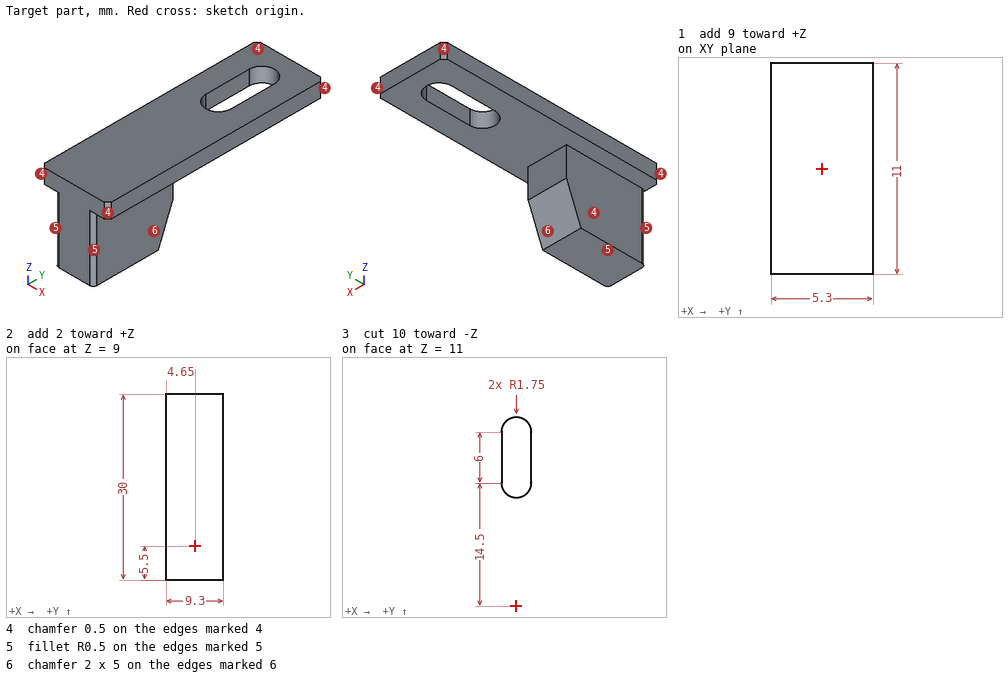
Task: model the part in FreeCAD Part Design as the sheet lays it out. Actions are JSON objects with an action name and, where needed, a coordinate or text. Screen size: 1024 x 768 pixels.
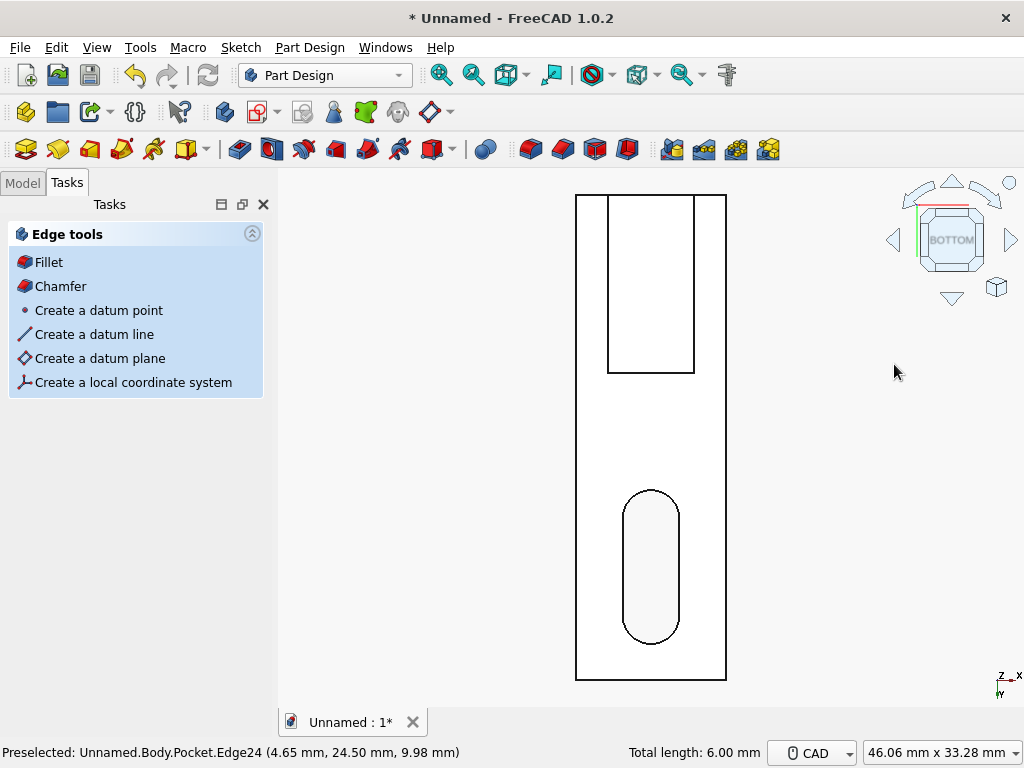
{"action": "key", "text": "4"}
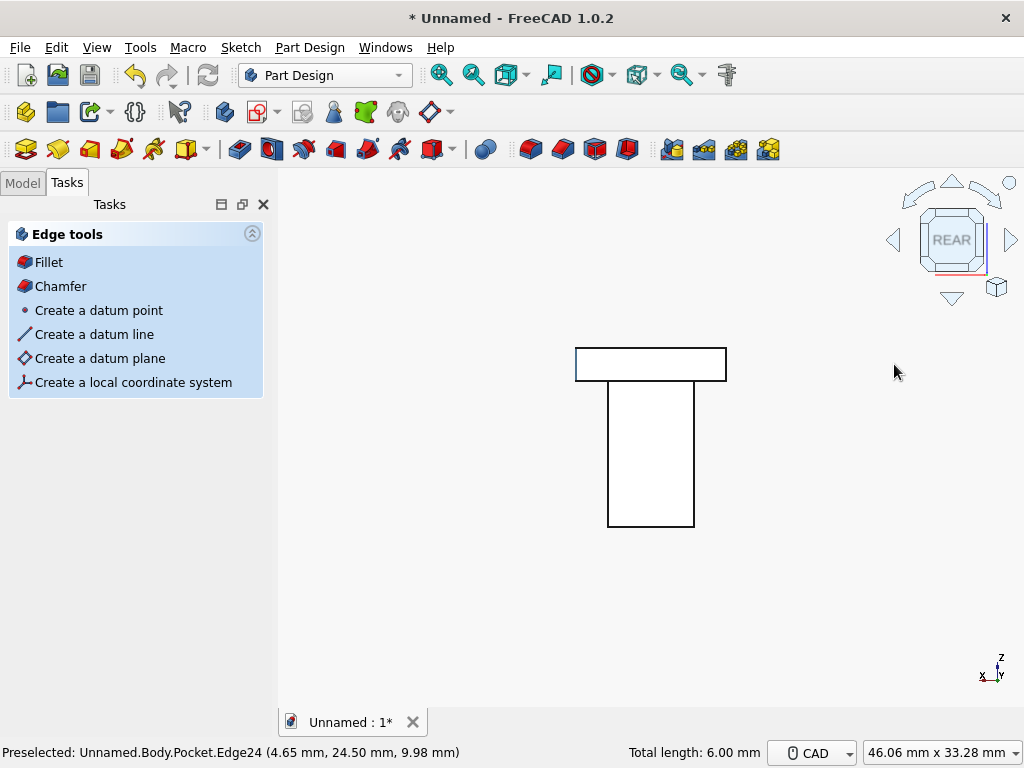
{"action": "left_click", "coordinate": [442, 76]}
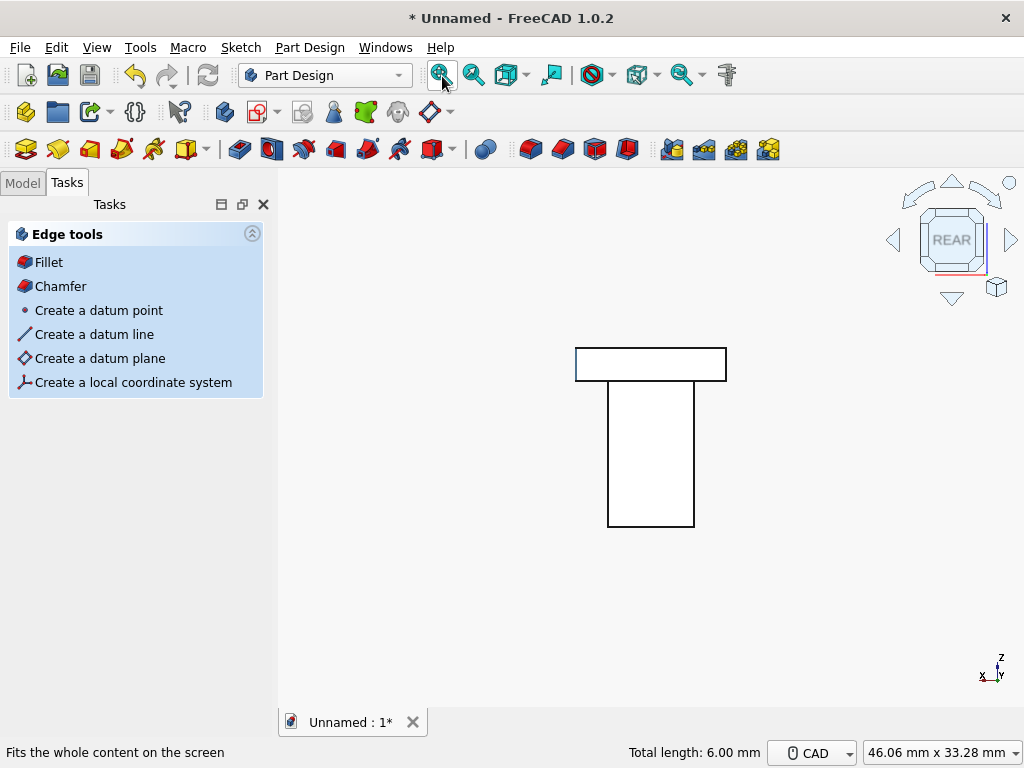
{"action": "left_click", "coordinate": [726, 364], "text": "ctrl"}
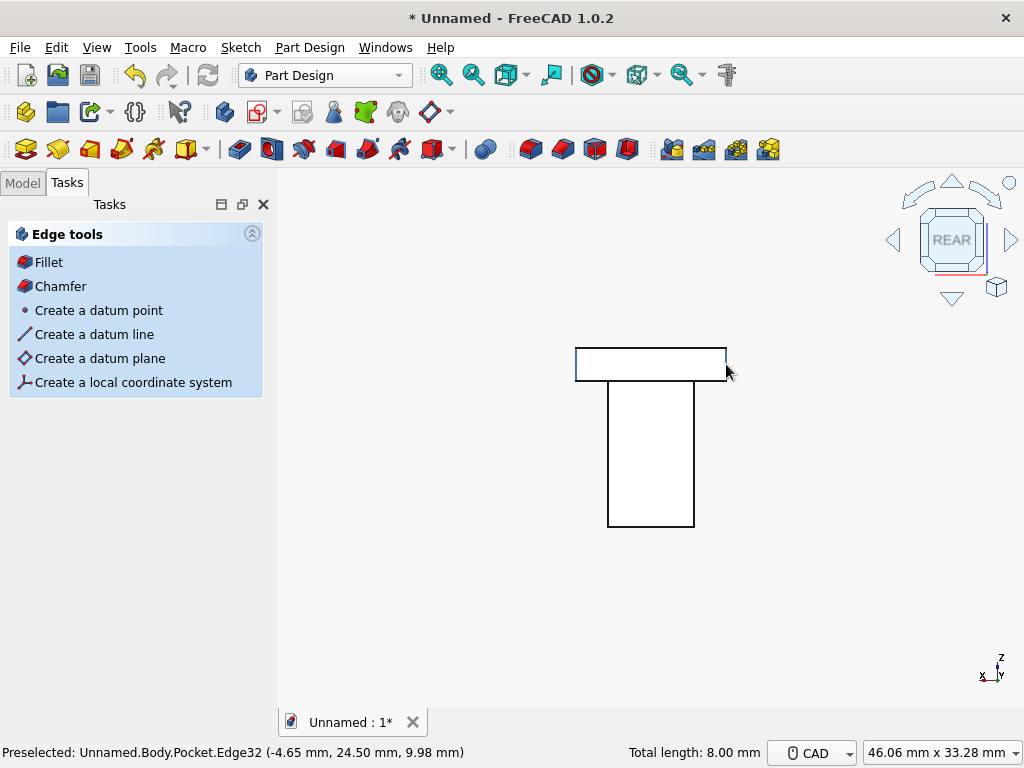
{"action": "left_click", "coordinate": [564, 150]}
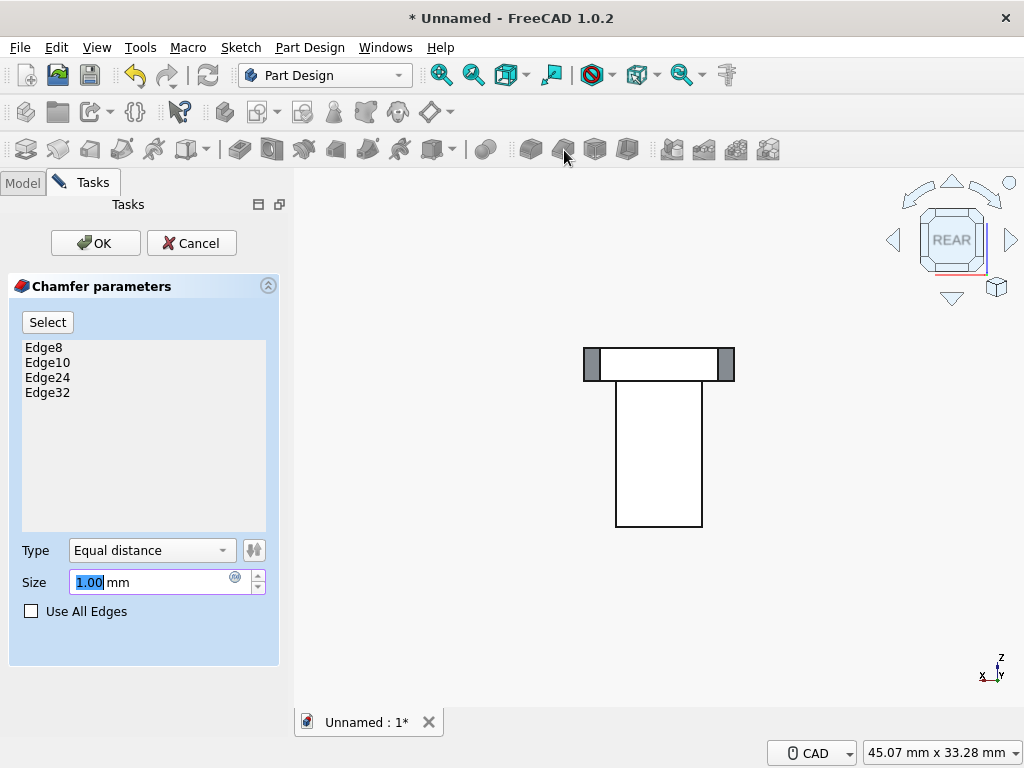
{"action": "type", "text": "0.5"}
{"action": "key", "text": "Tab"}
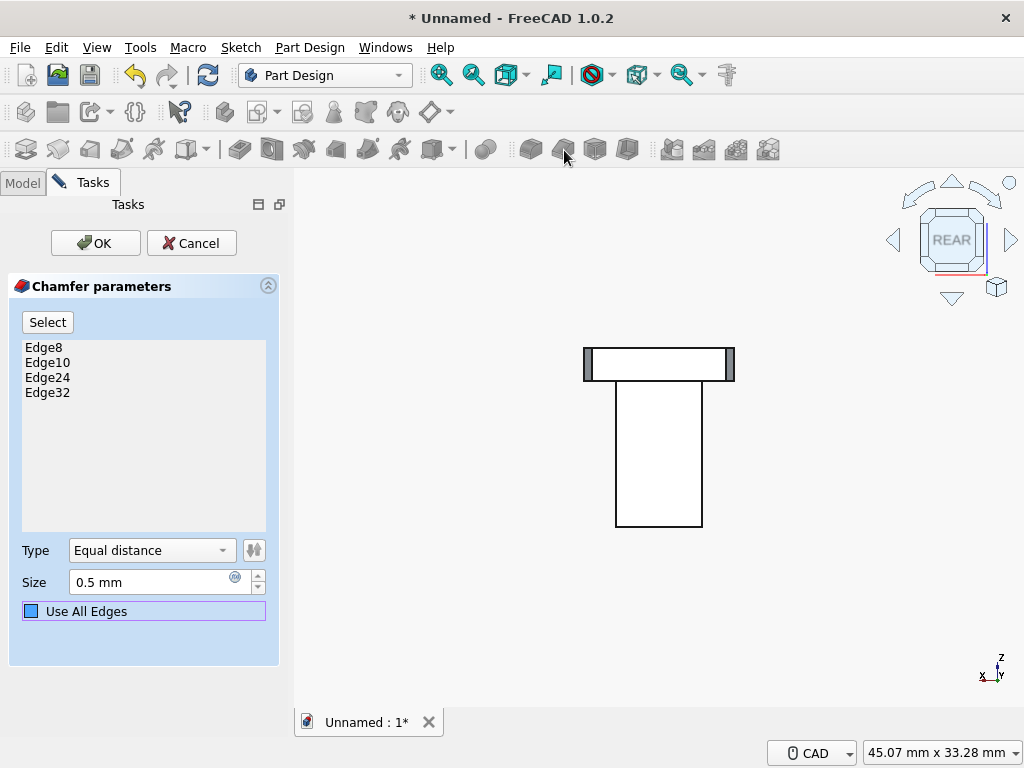
{"action": "left_click", "coordinate": [96, 243]}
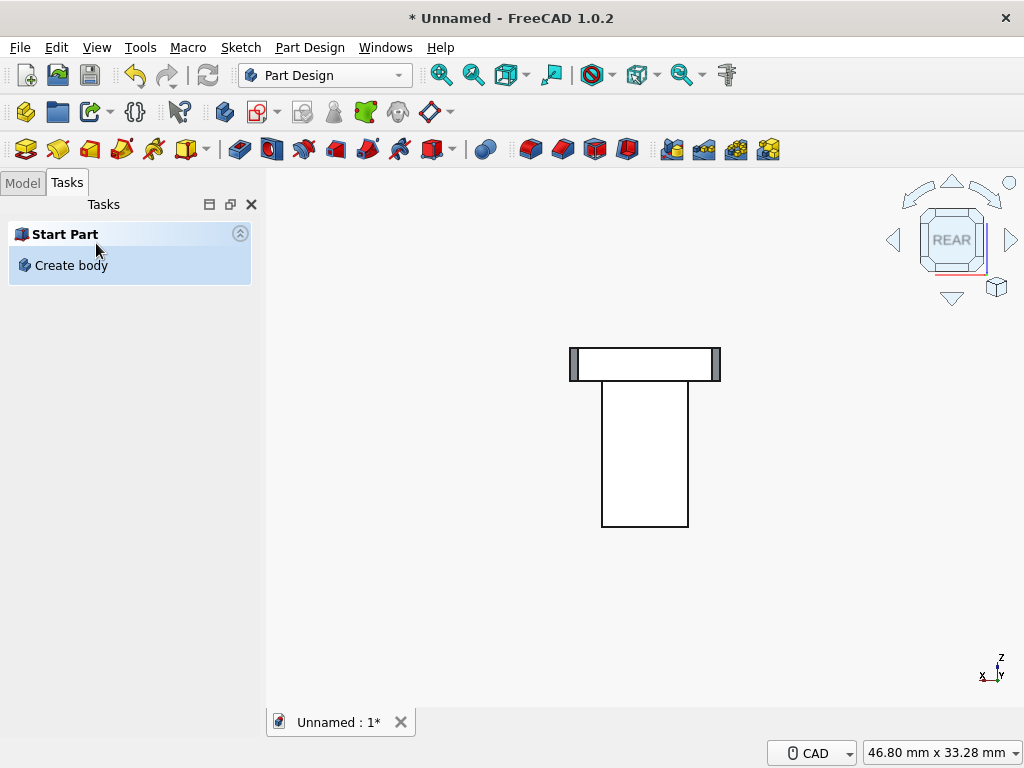
{"action": "left_click", "coordinate": [442, 76]}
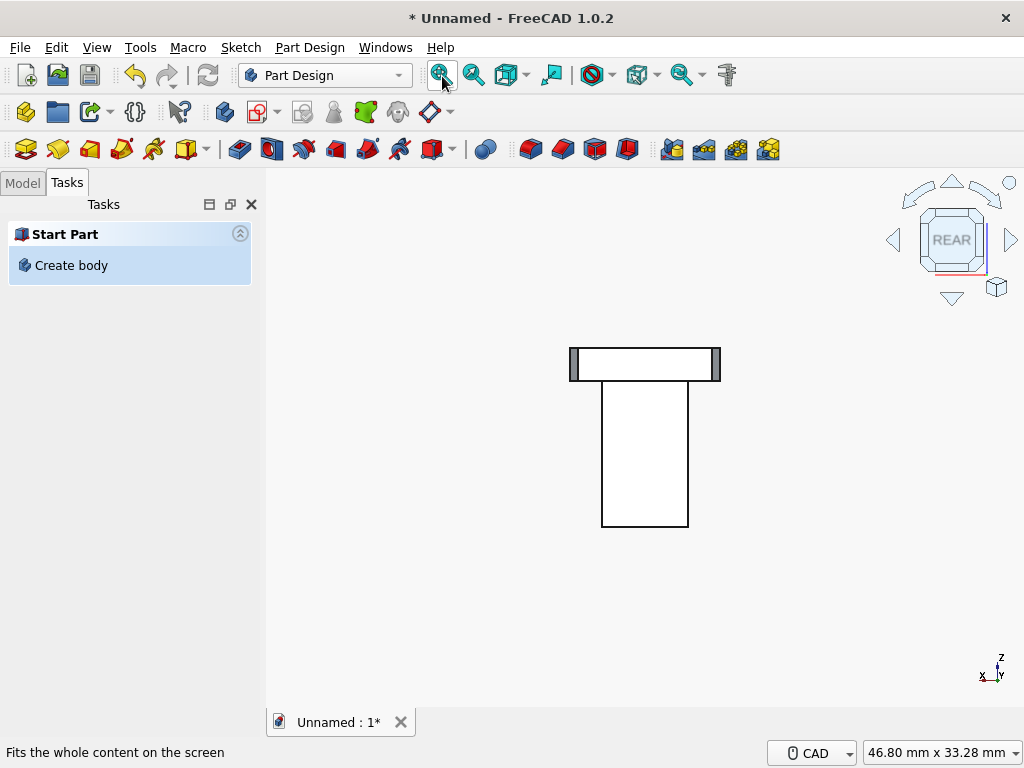
{"action": "key", "text": "0"}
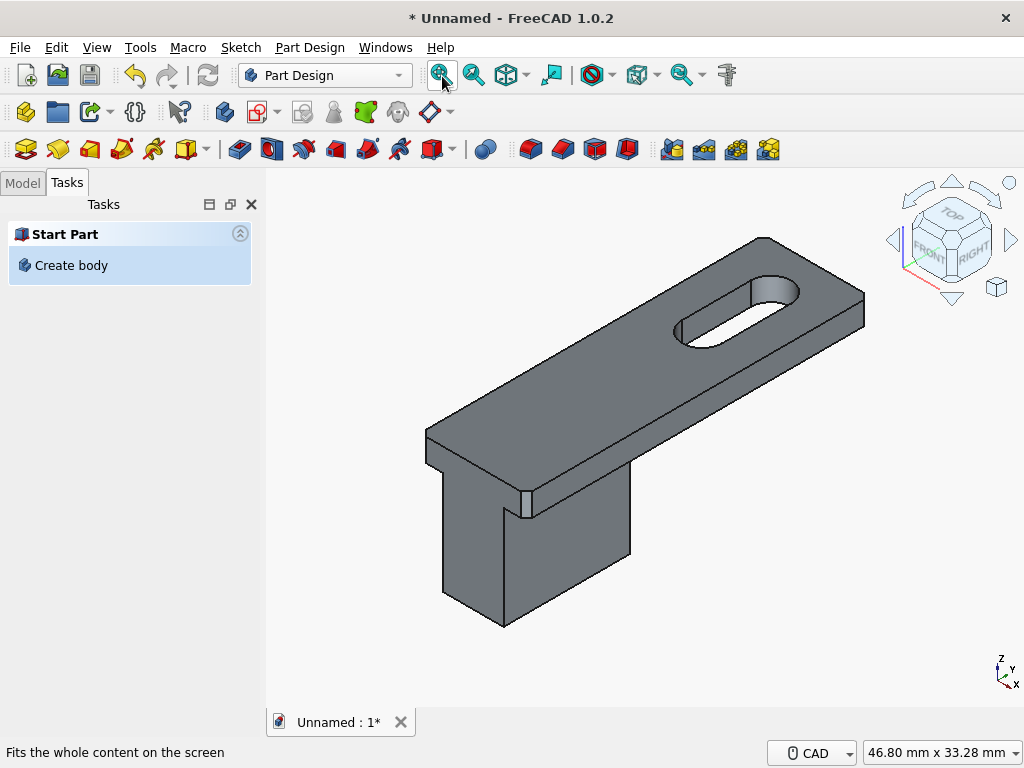
{"action": "left_click", "coordinate": [504, 566]}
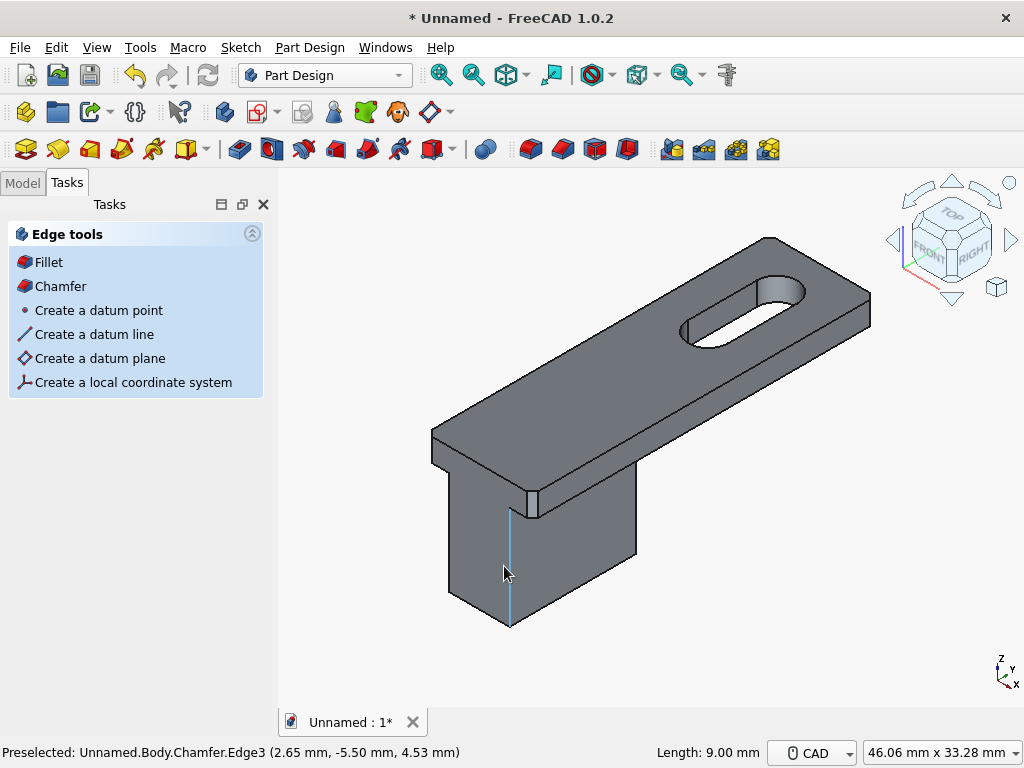
{"action": "key", "text": "2"}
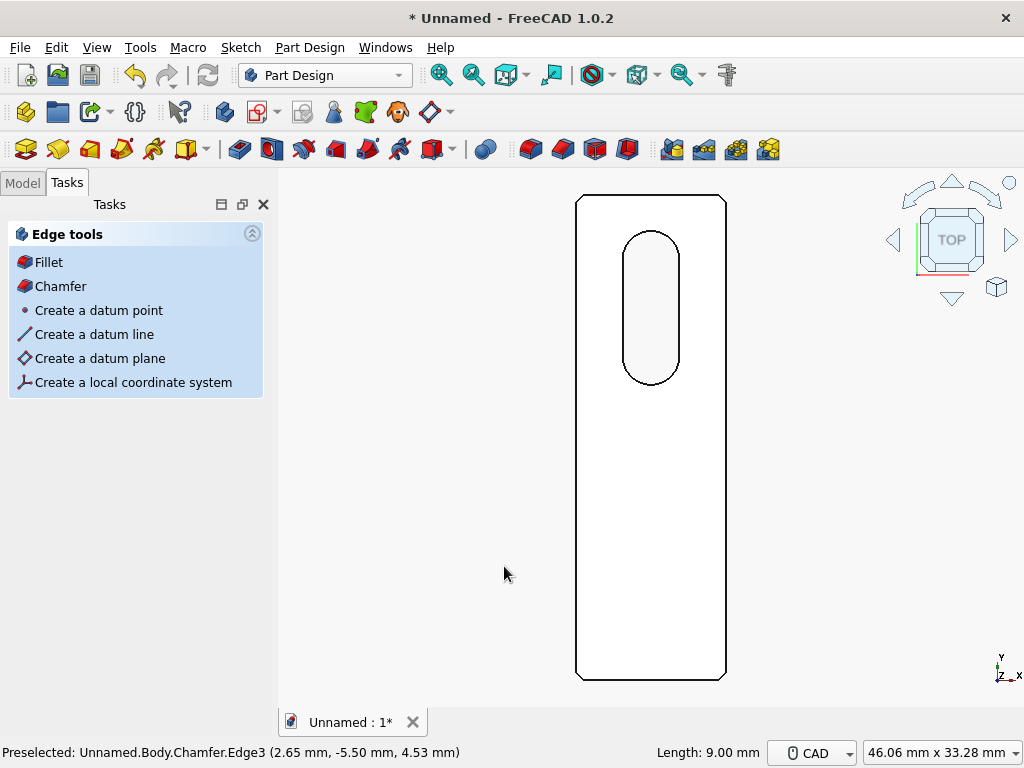
{"action": "key", "text": "1"}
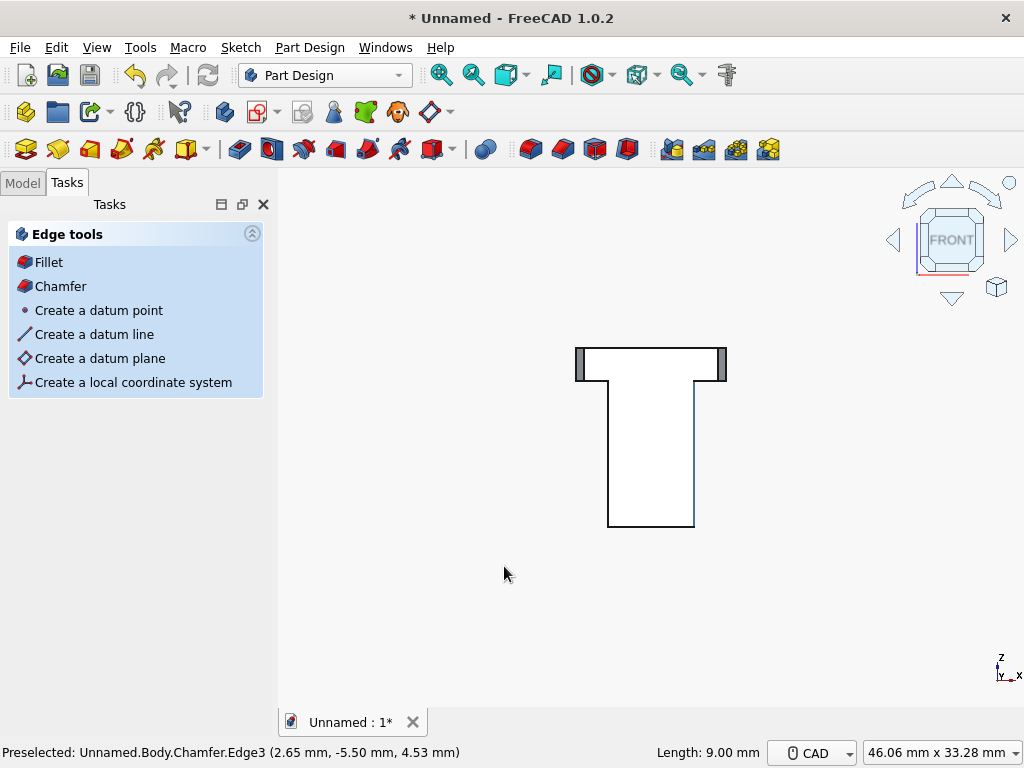
{"action": "left_click", "coordinate": [442, 76]}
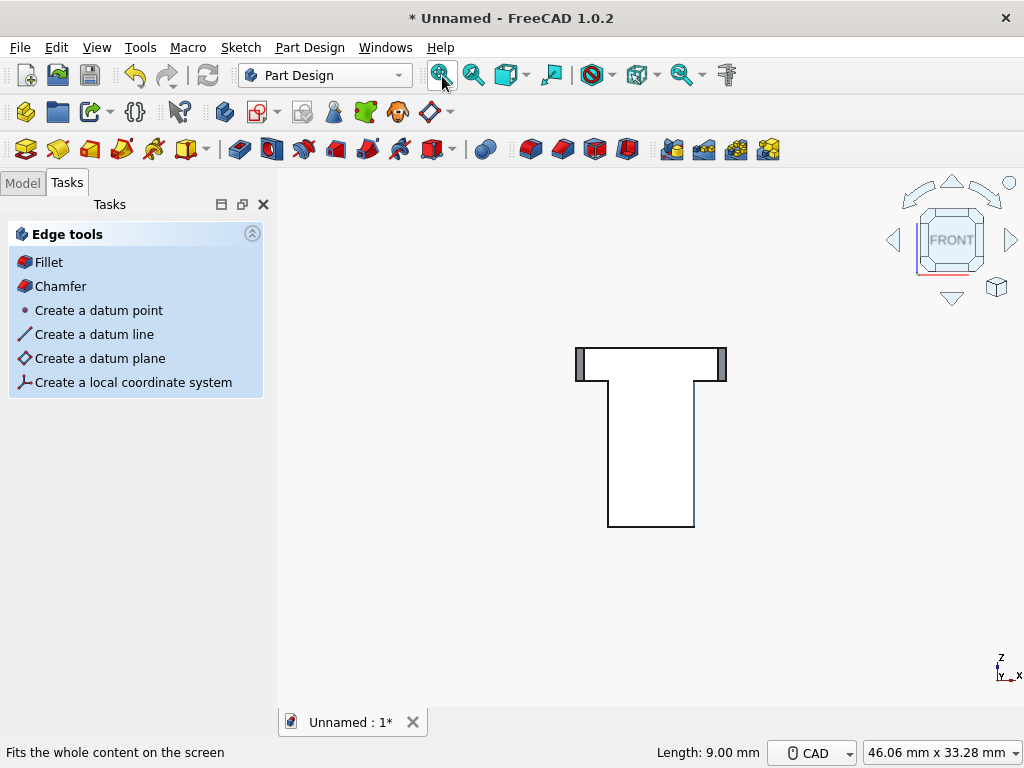
{"action": "left_click", "coordinate": [608, 453], "text": "ctrl"}